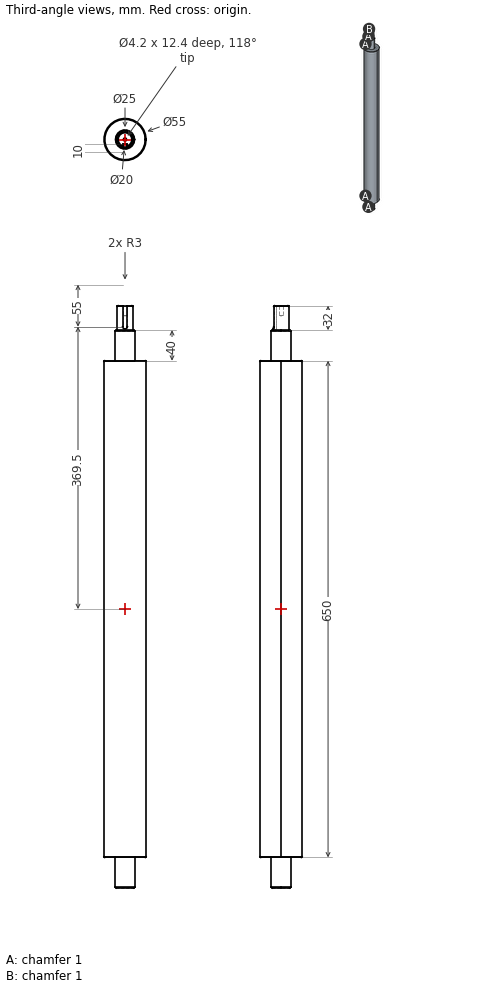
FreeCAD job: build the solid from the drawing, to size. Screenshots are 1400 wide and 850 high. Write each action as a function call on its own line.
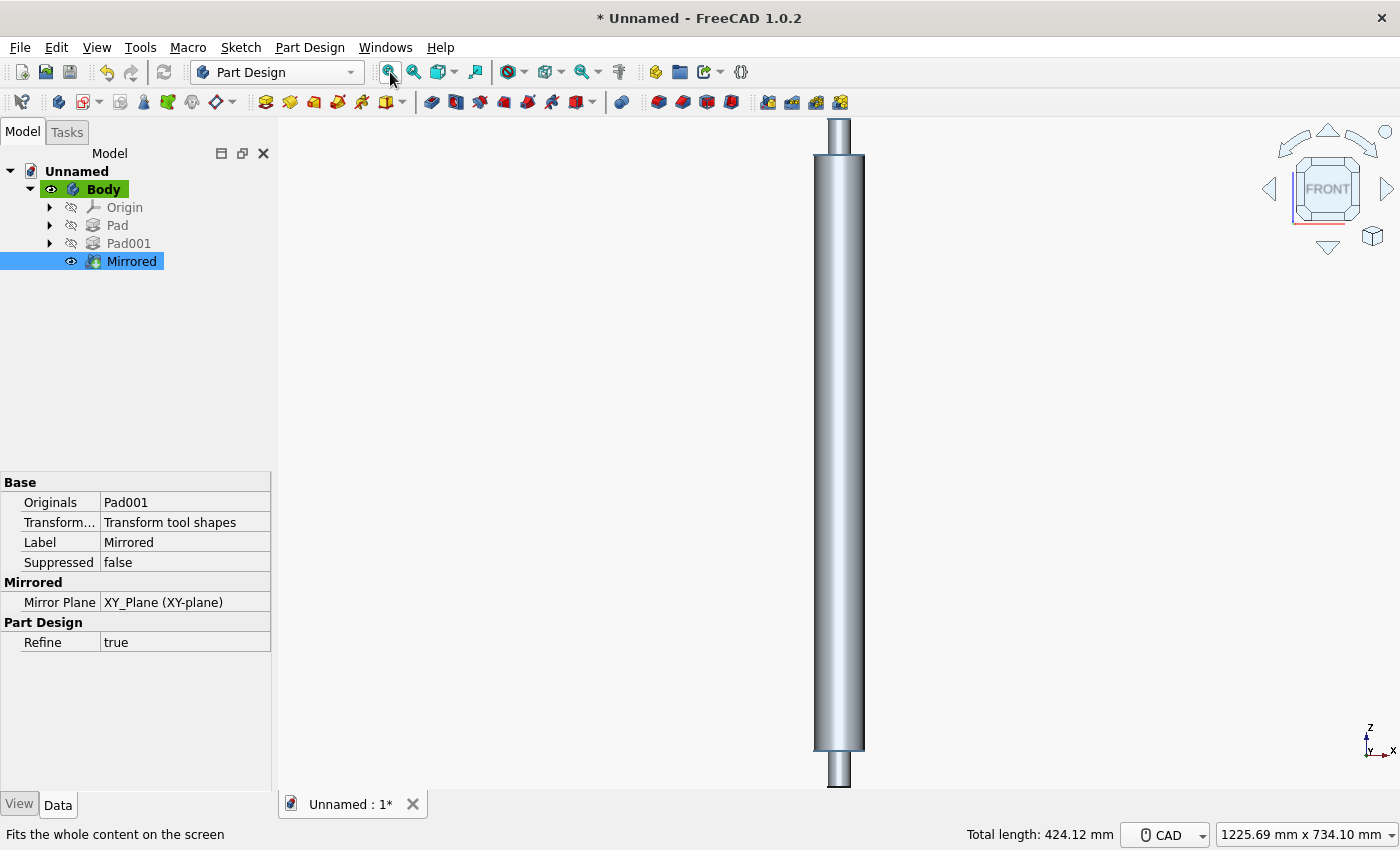
key(3)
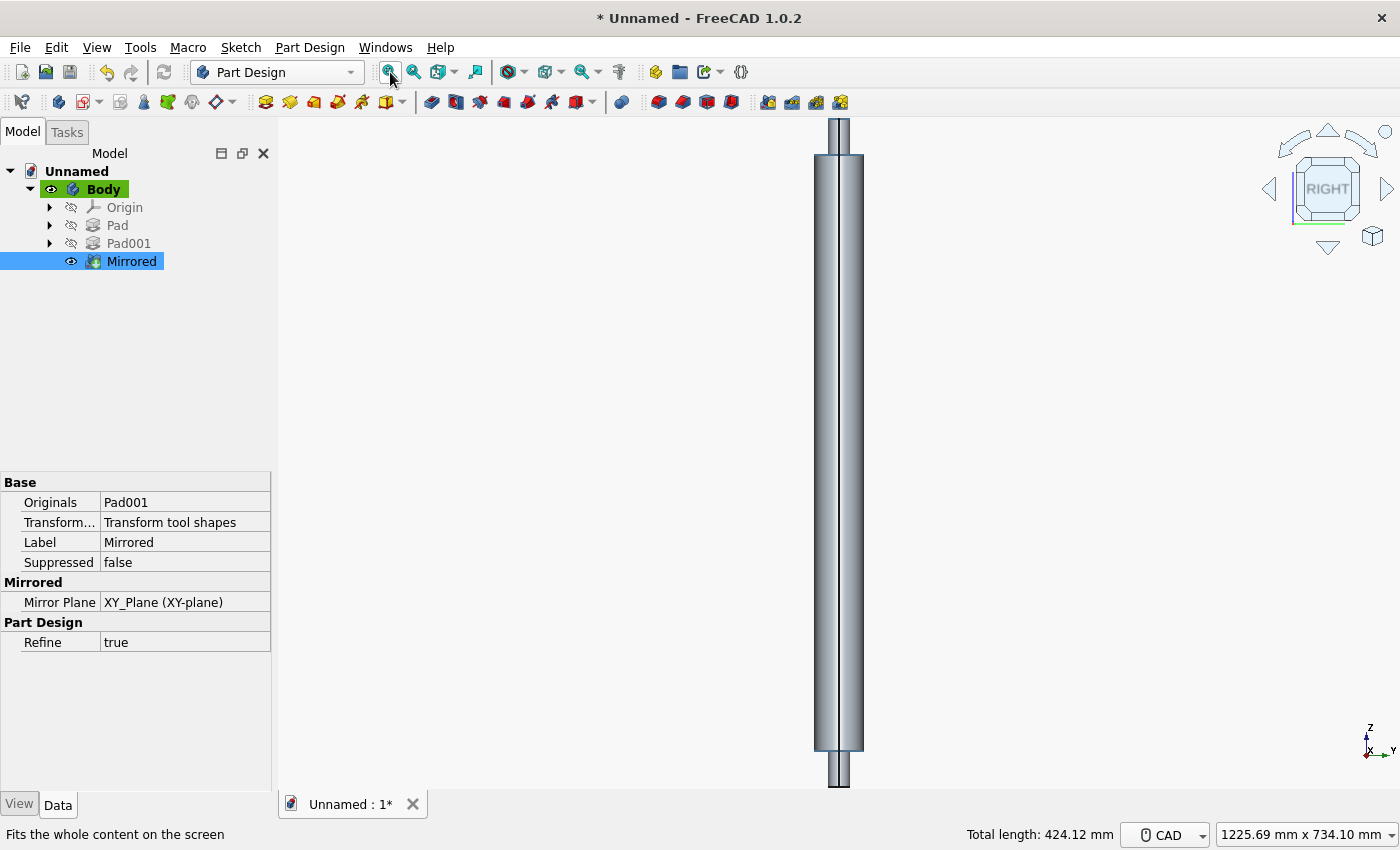
key(5)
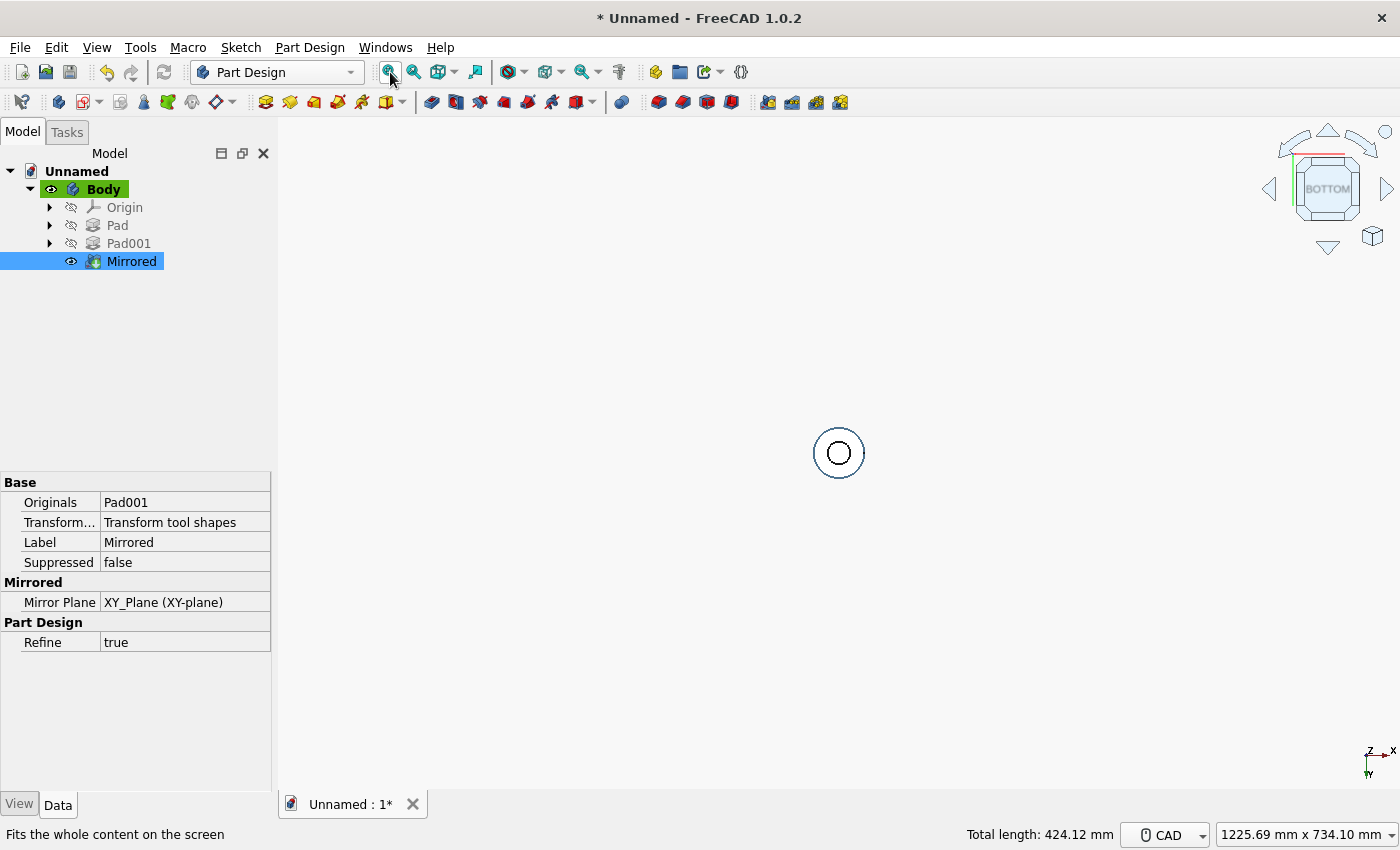
key(v)
key(f)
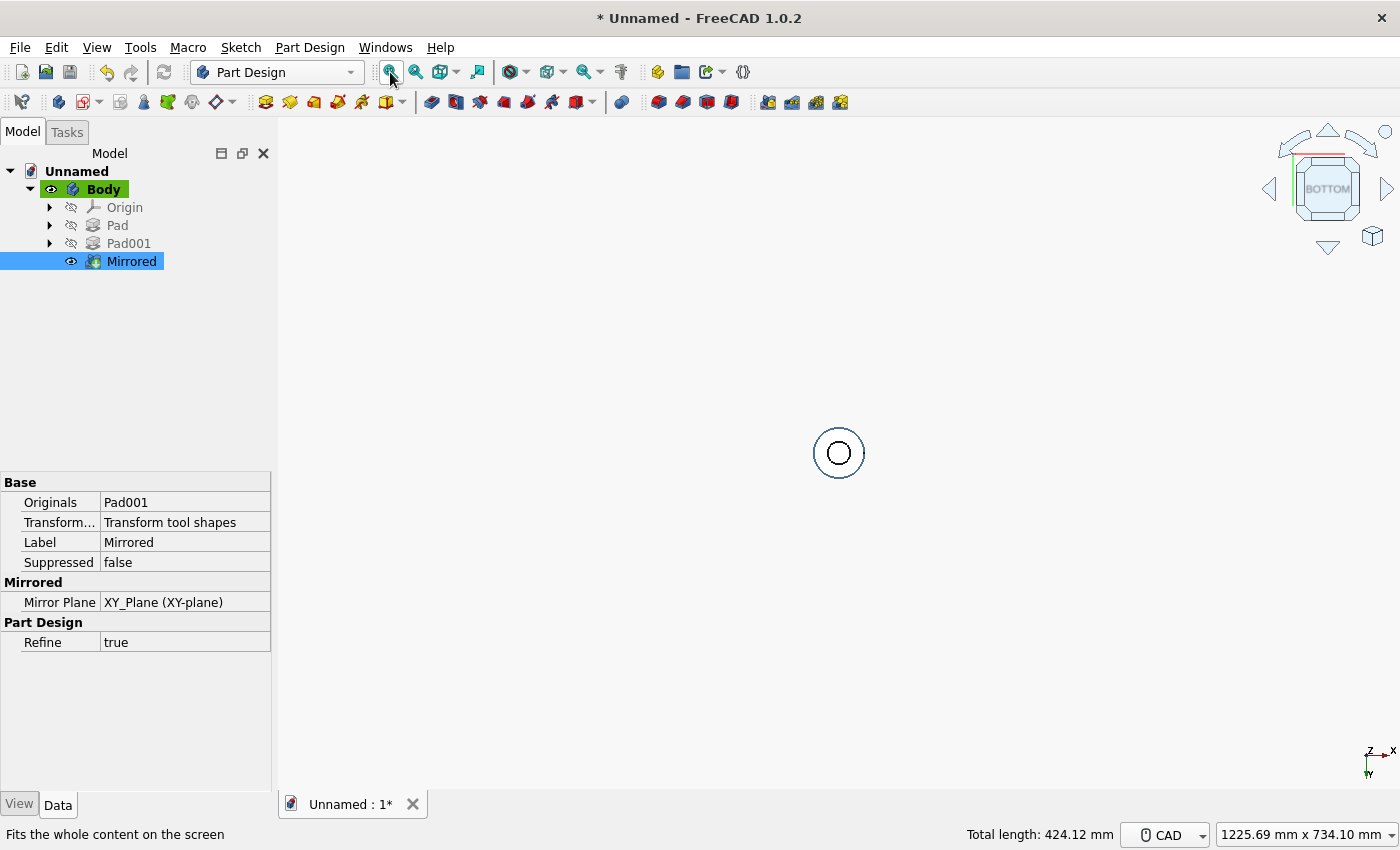
click(828, 452, ctrl)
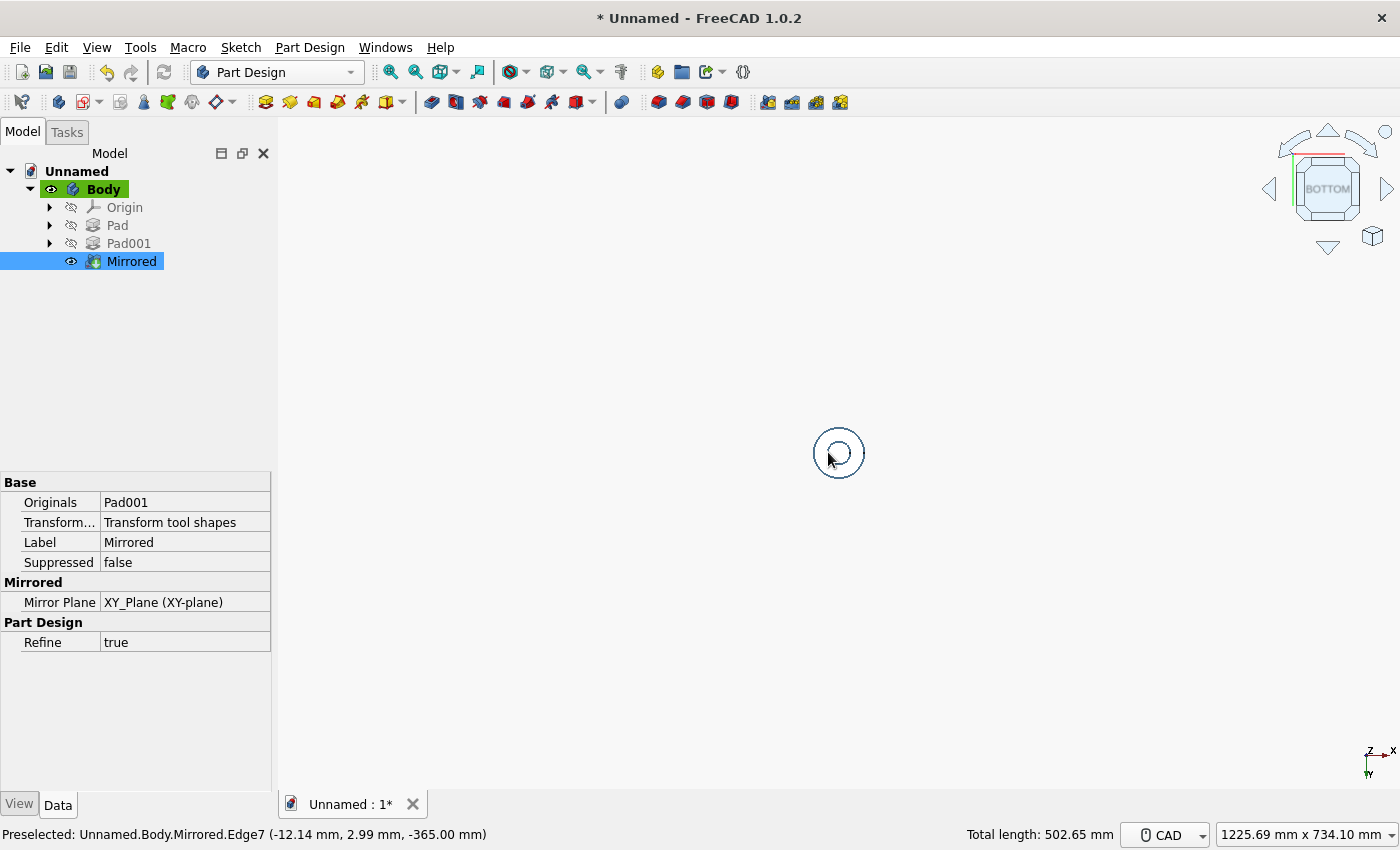
click(684, 102)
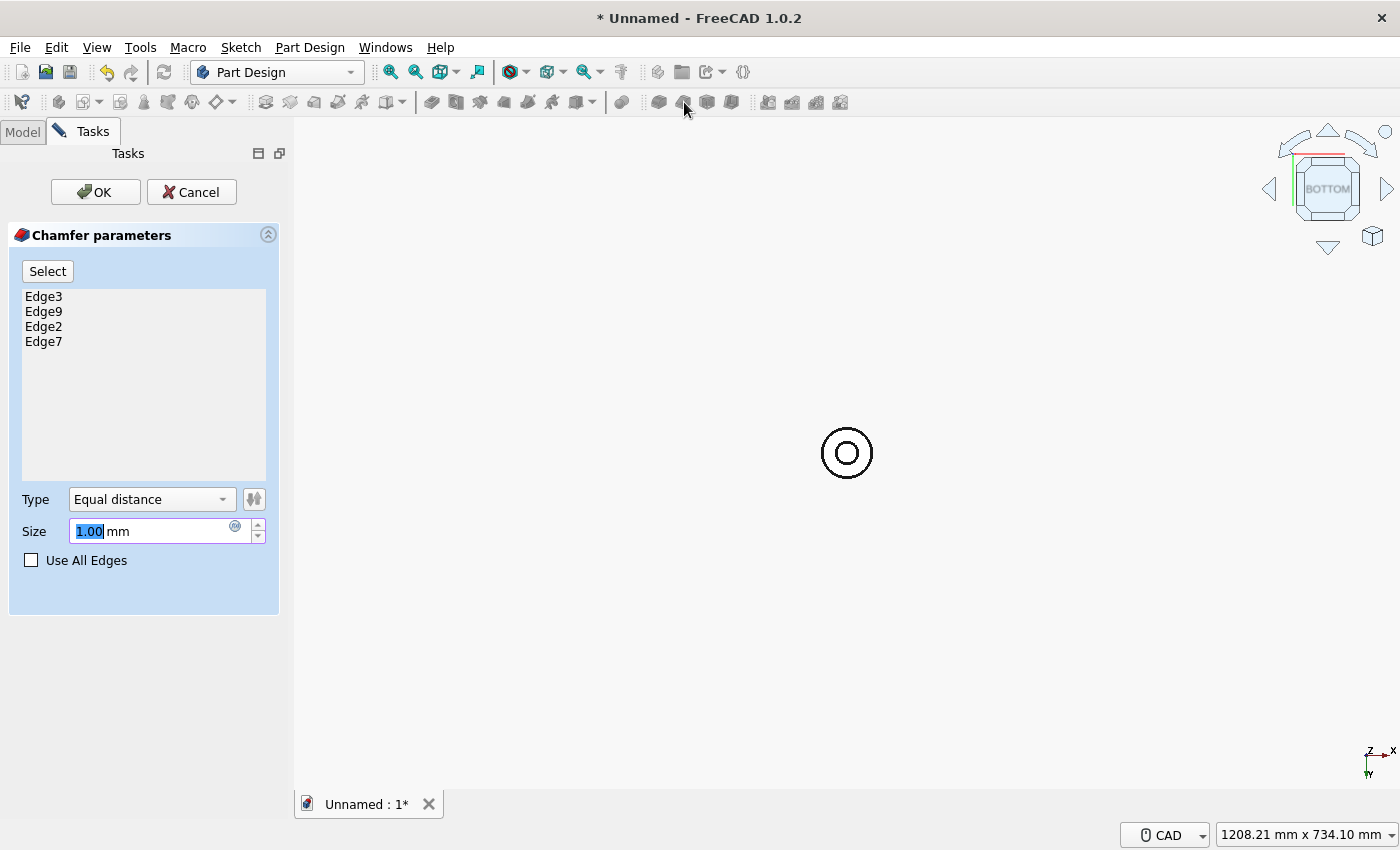
text(1)
key(Tab)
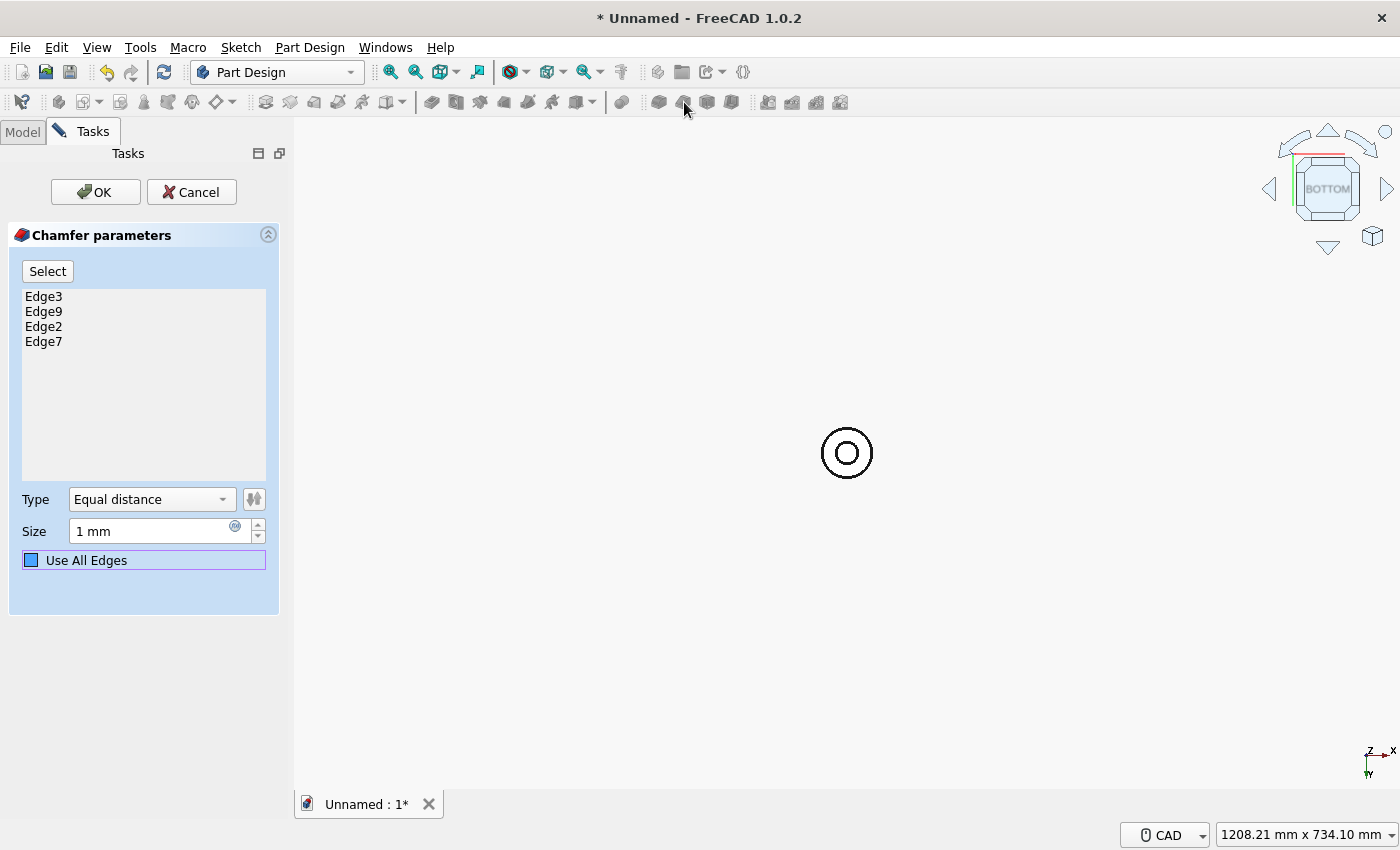
click(96, 192)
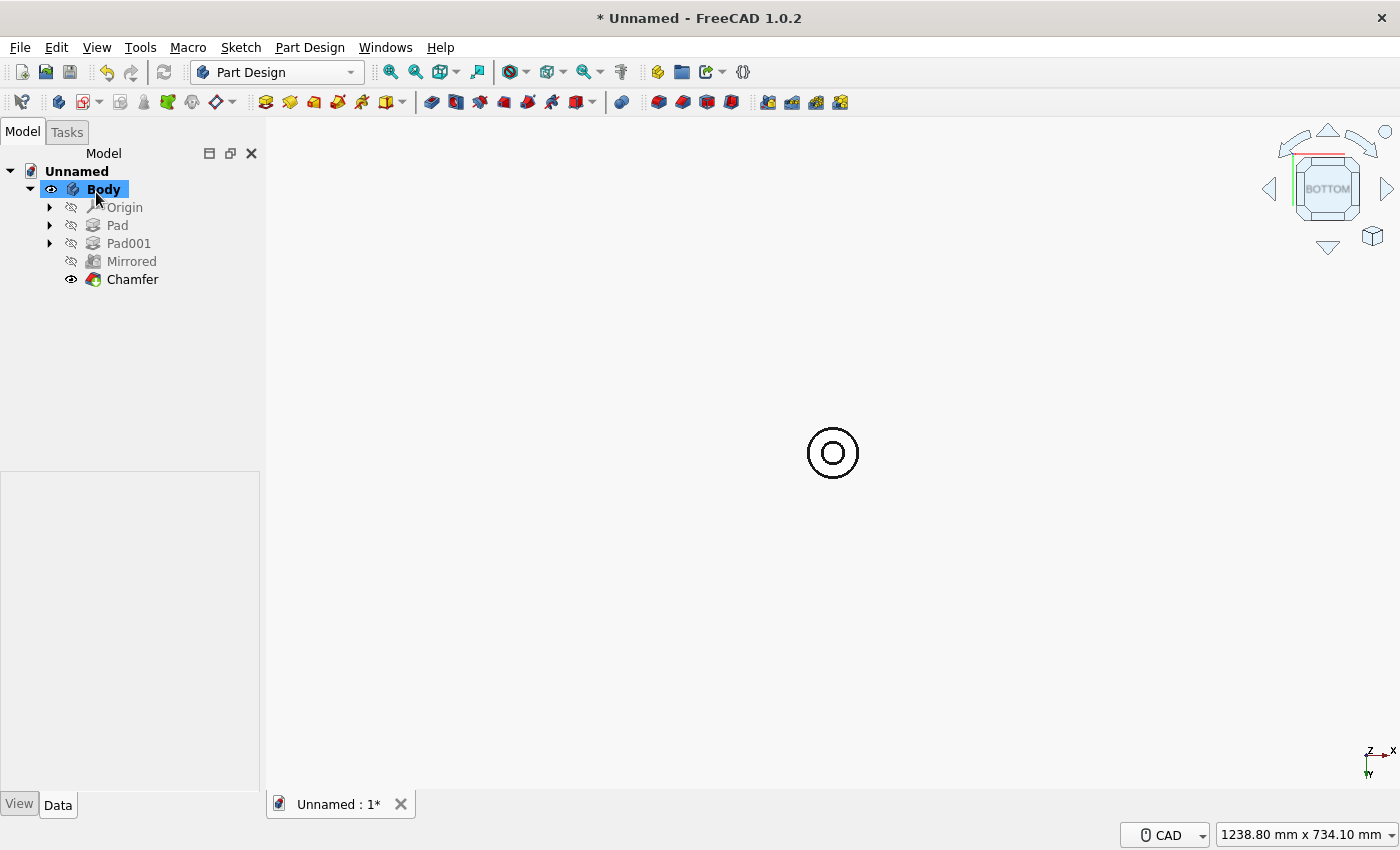
click(392, 72)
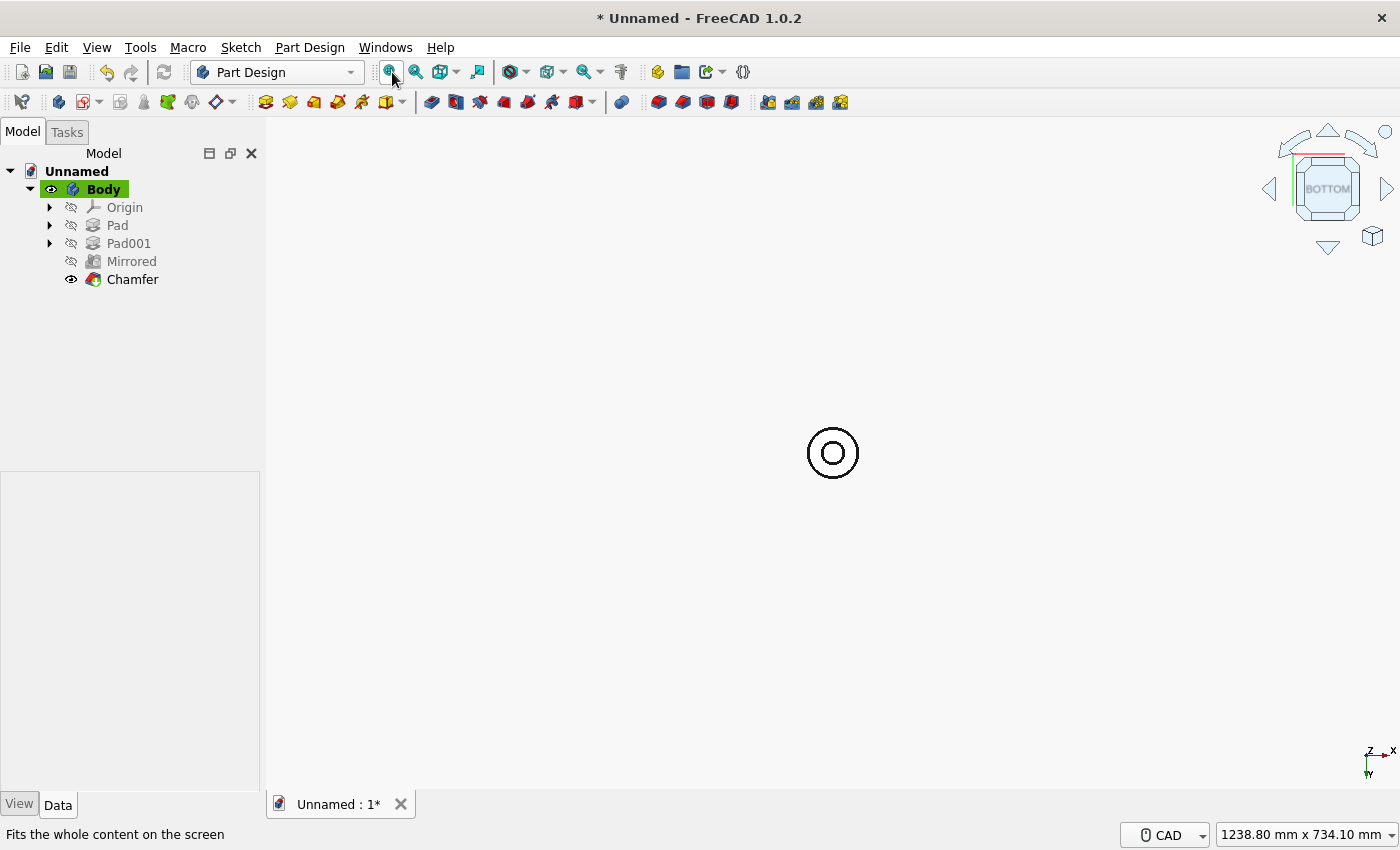
key(0)